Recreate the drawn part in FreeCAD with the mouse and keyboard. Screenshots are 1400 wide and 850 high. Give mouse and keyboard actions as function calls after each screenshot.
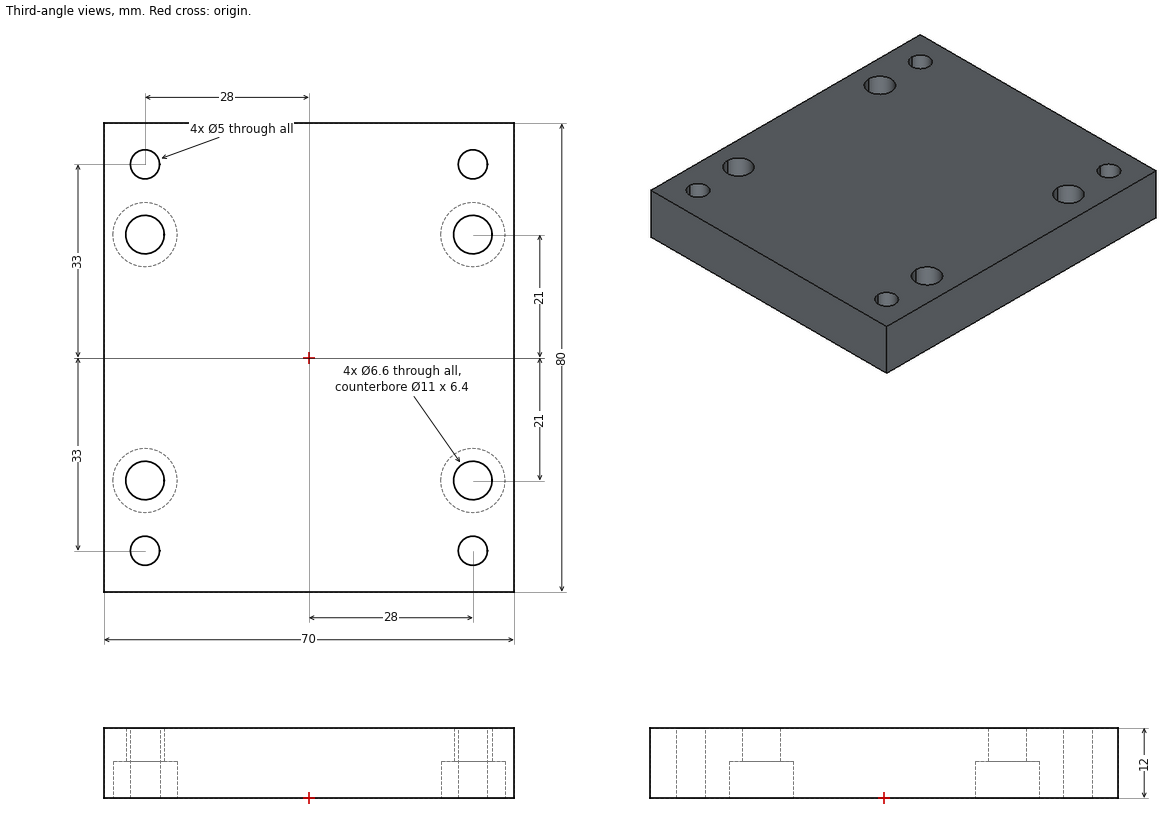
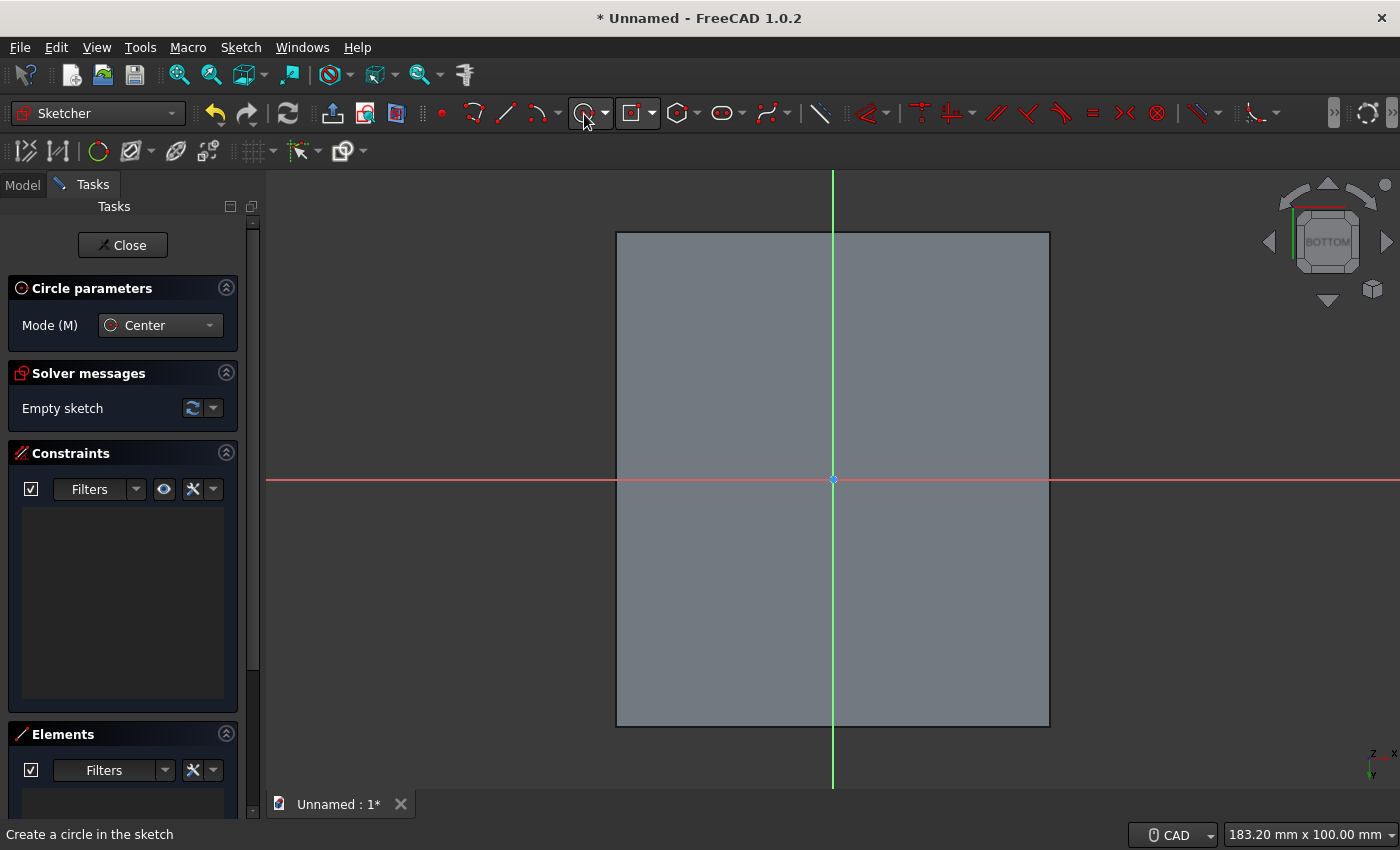
scroll(660, 684, up, 2)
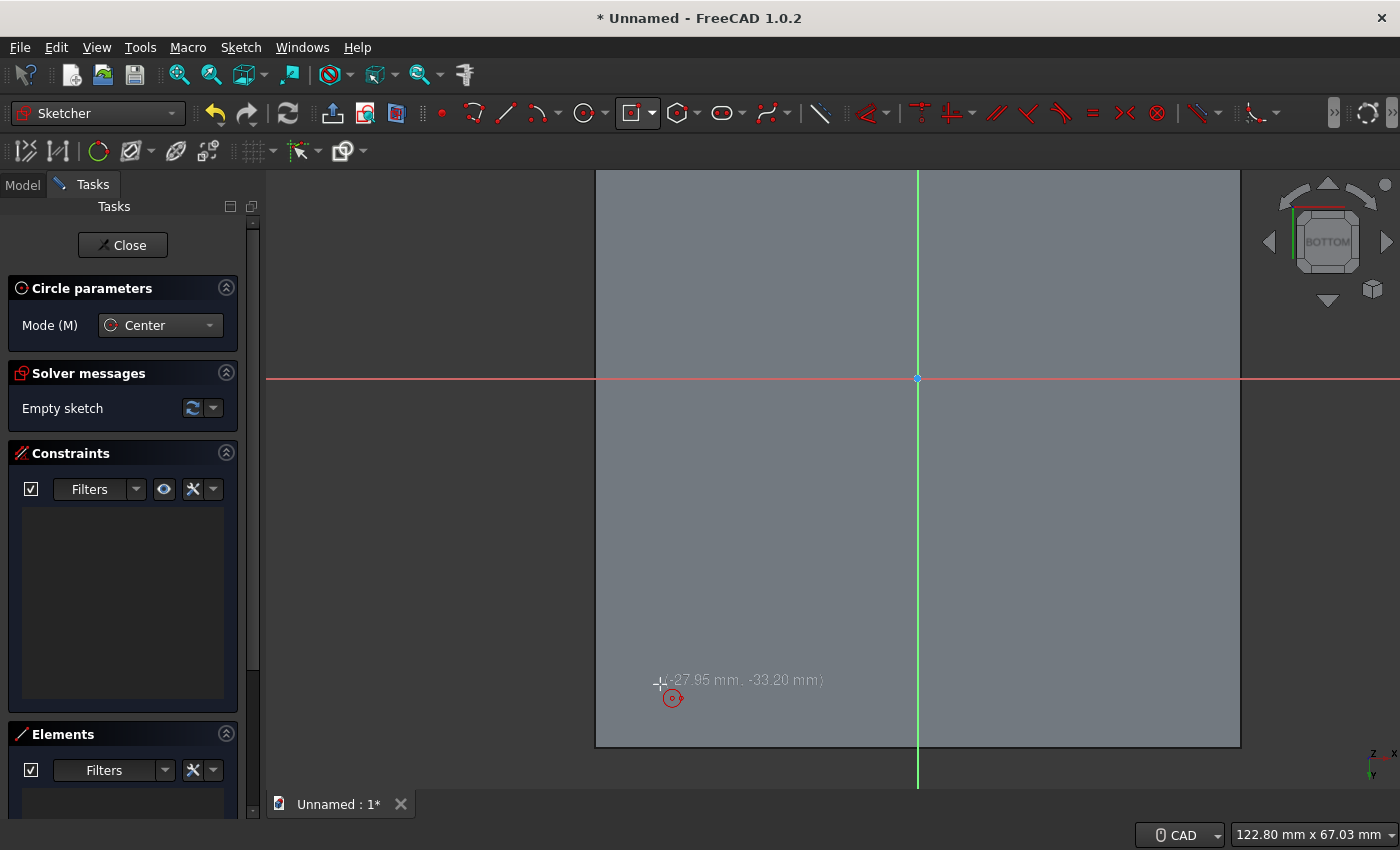
click(659, 683)
move(676, 667)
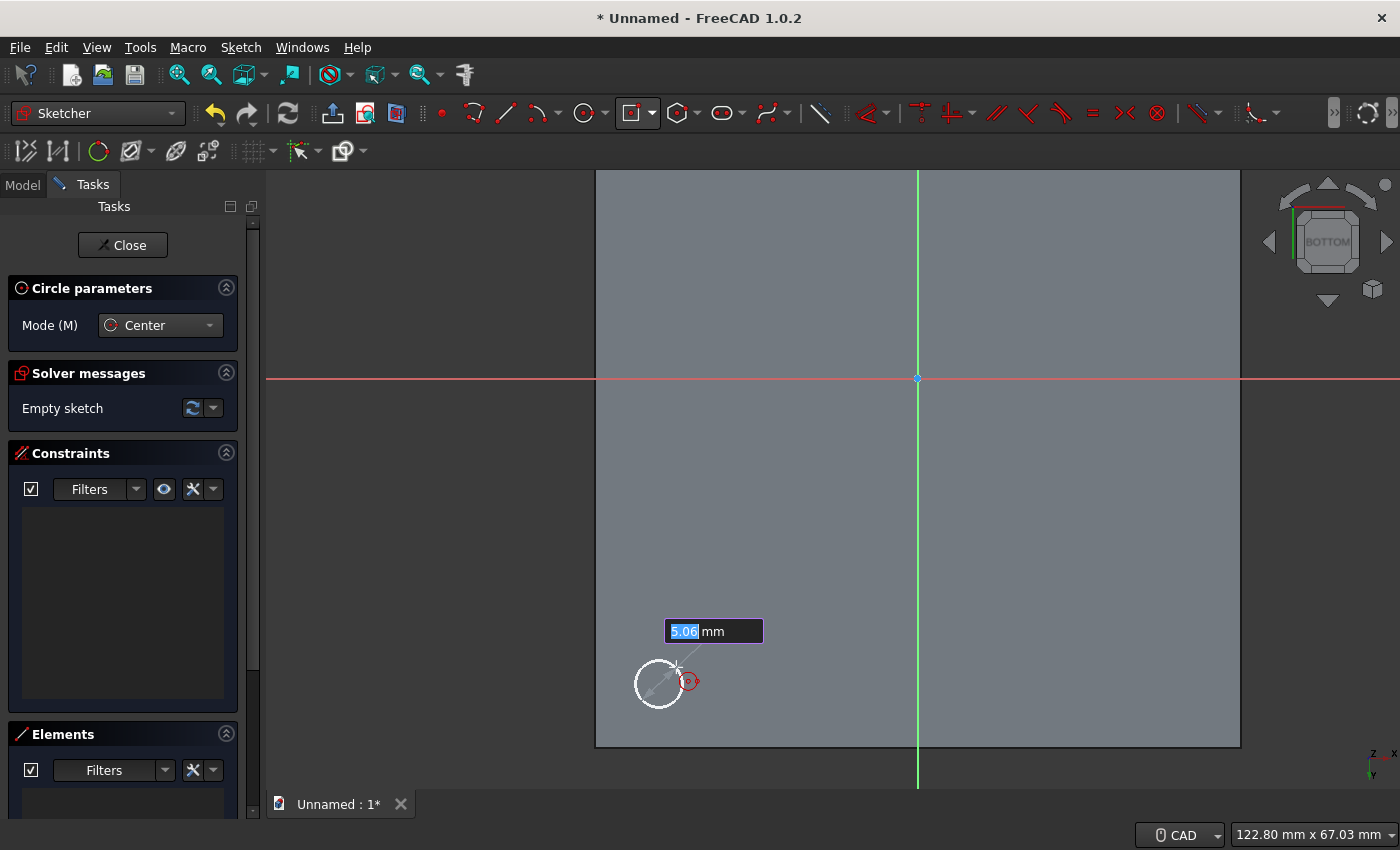
text(5)
key(Return)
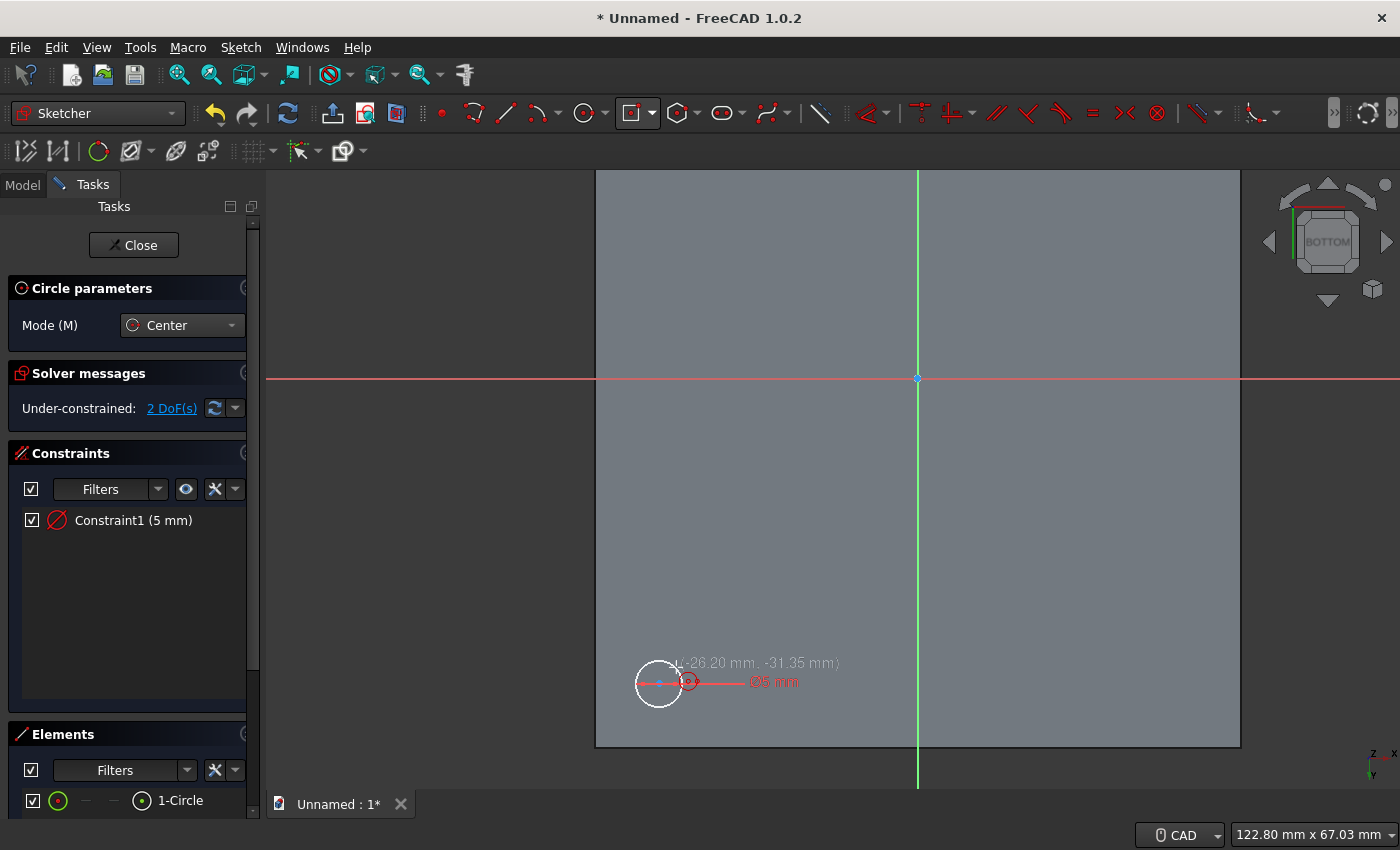
scroll(578, 602, down, 3)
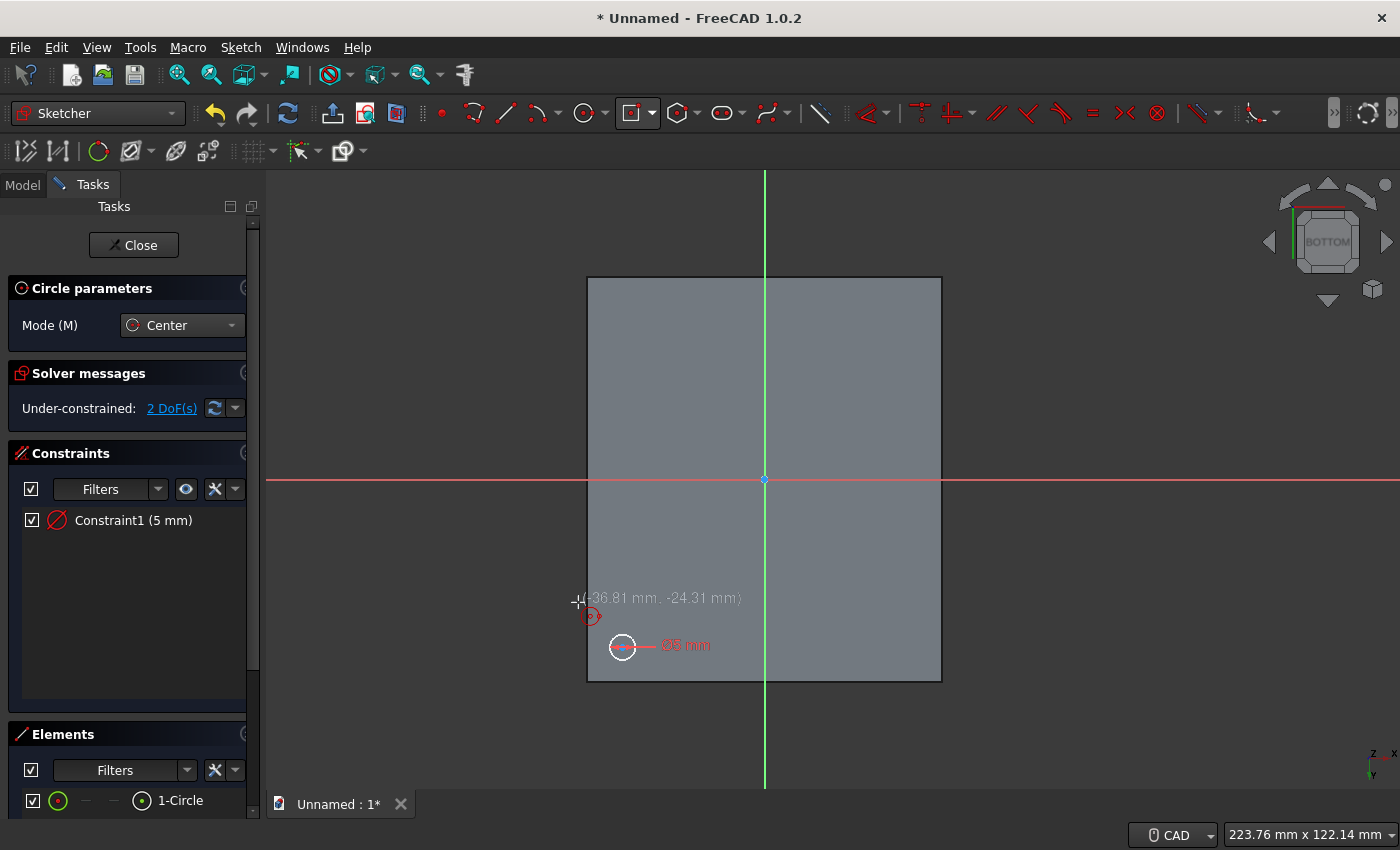
scroll(623, 312, up, 3)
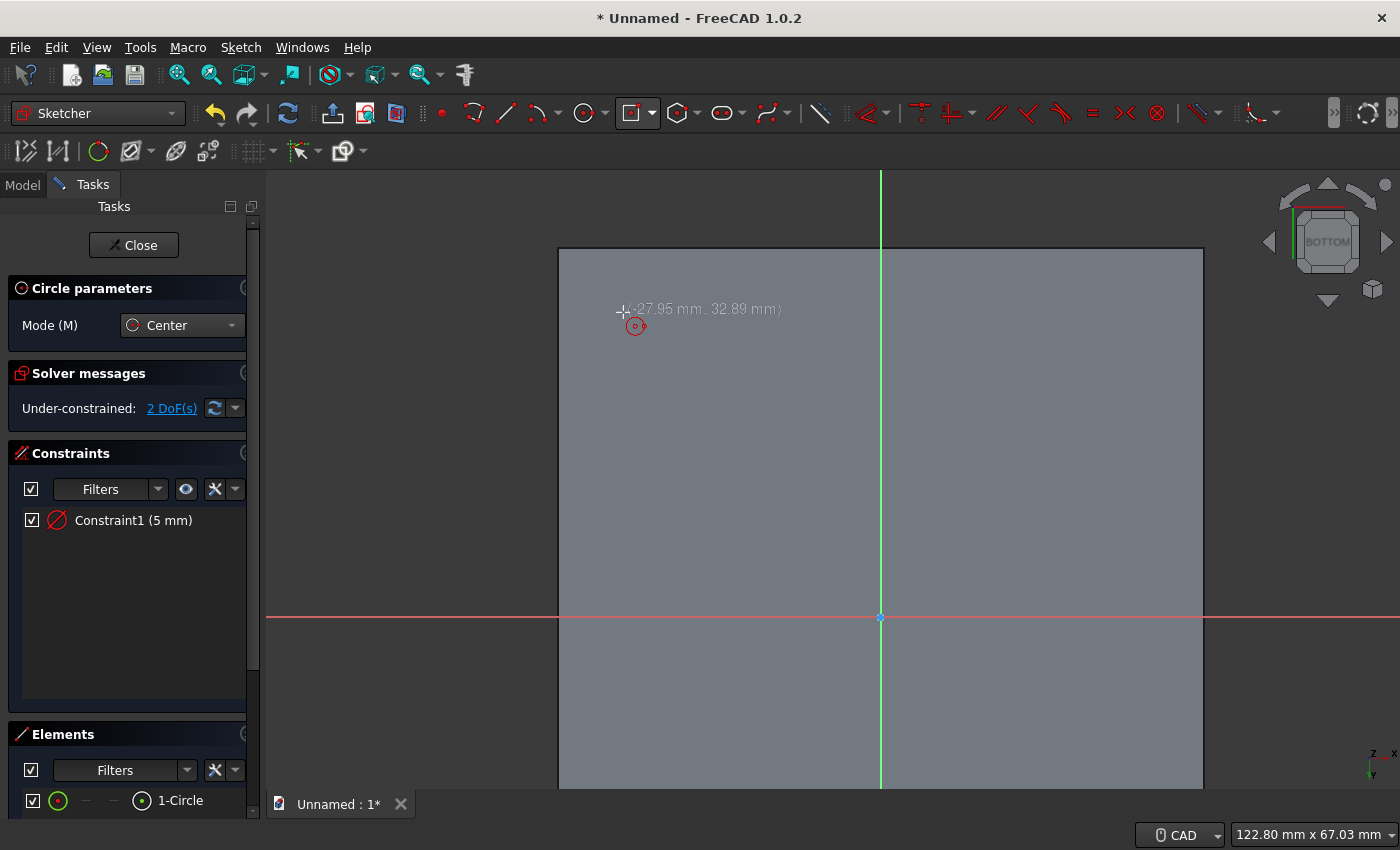
click(622, 313)
move(639, 296)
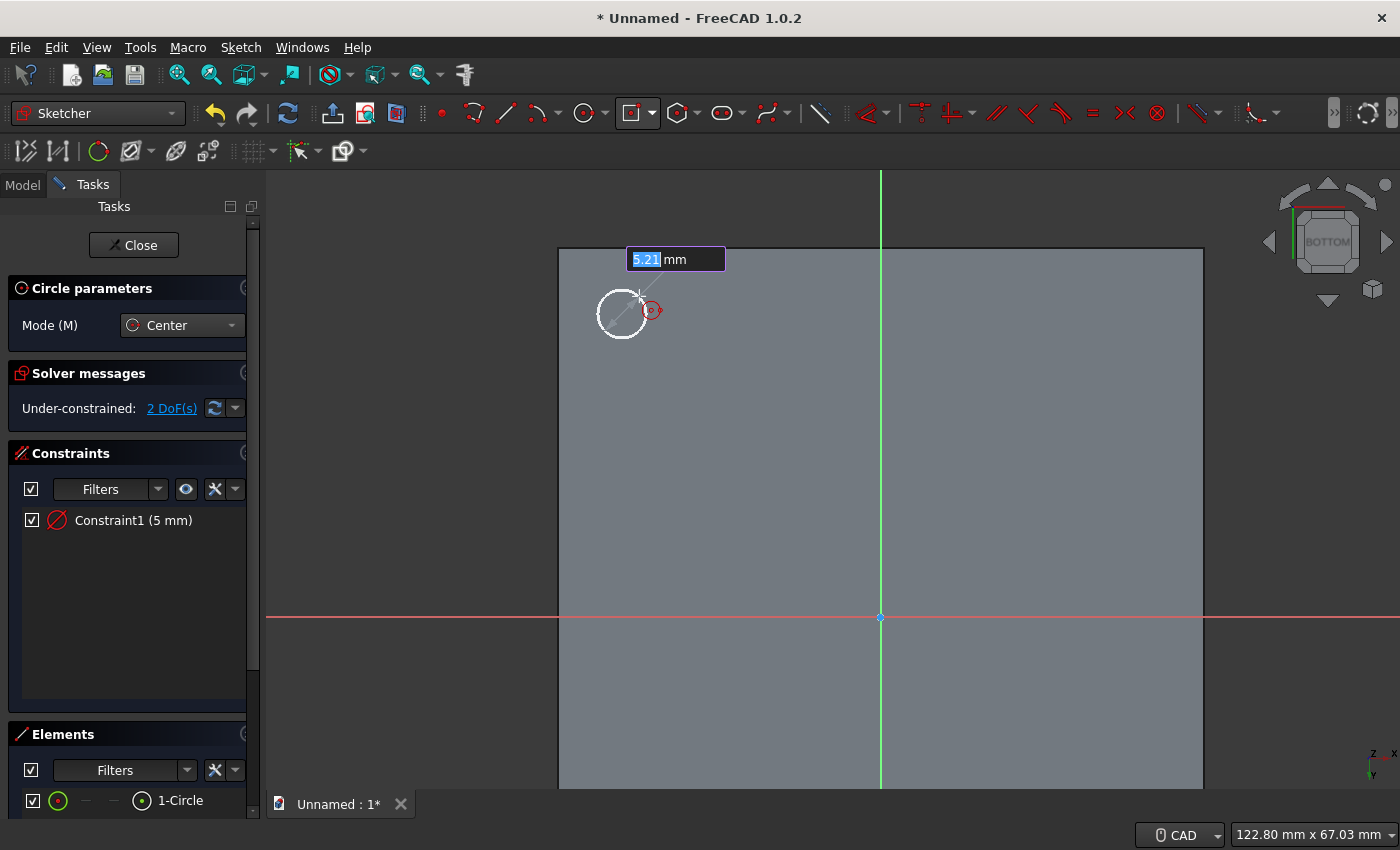
text(5)
key(Return)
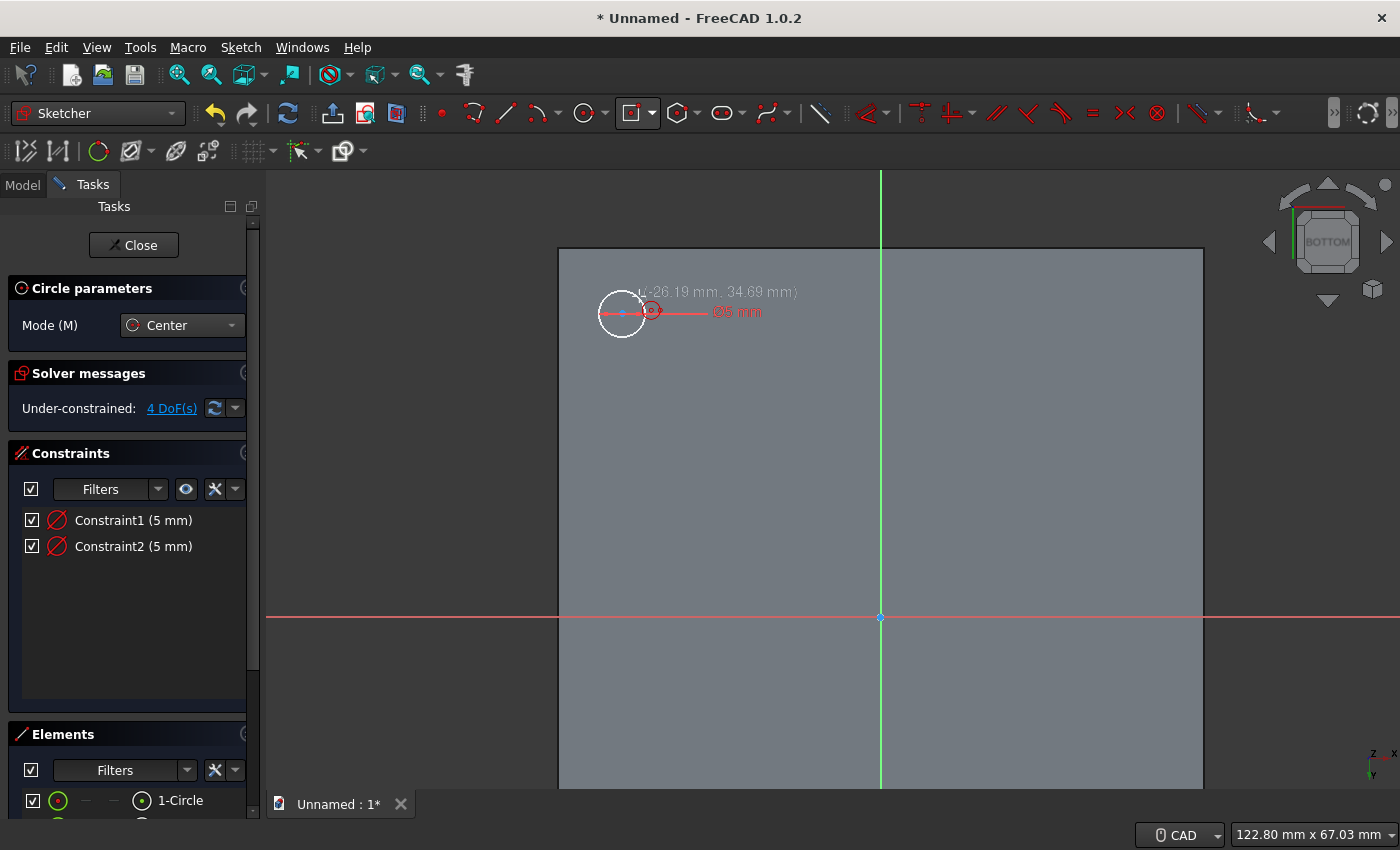
click(1139, 313)
move(1156, 296)